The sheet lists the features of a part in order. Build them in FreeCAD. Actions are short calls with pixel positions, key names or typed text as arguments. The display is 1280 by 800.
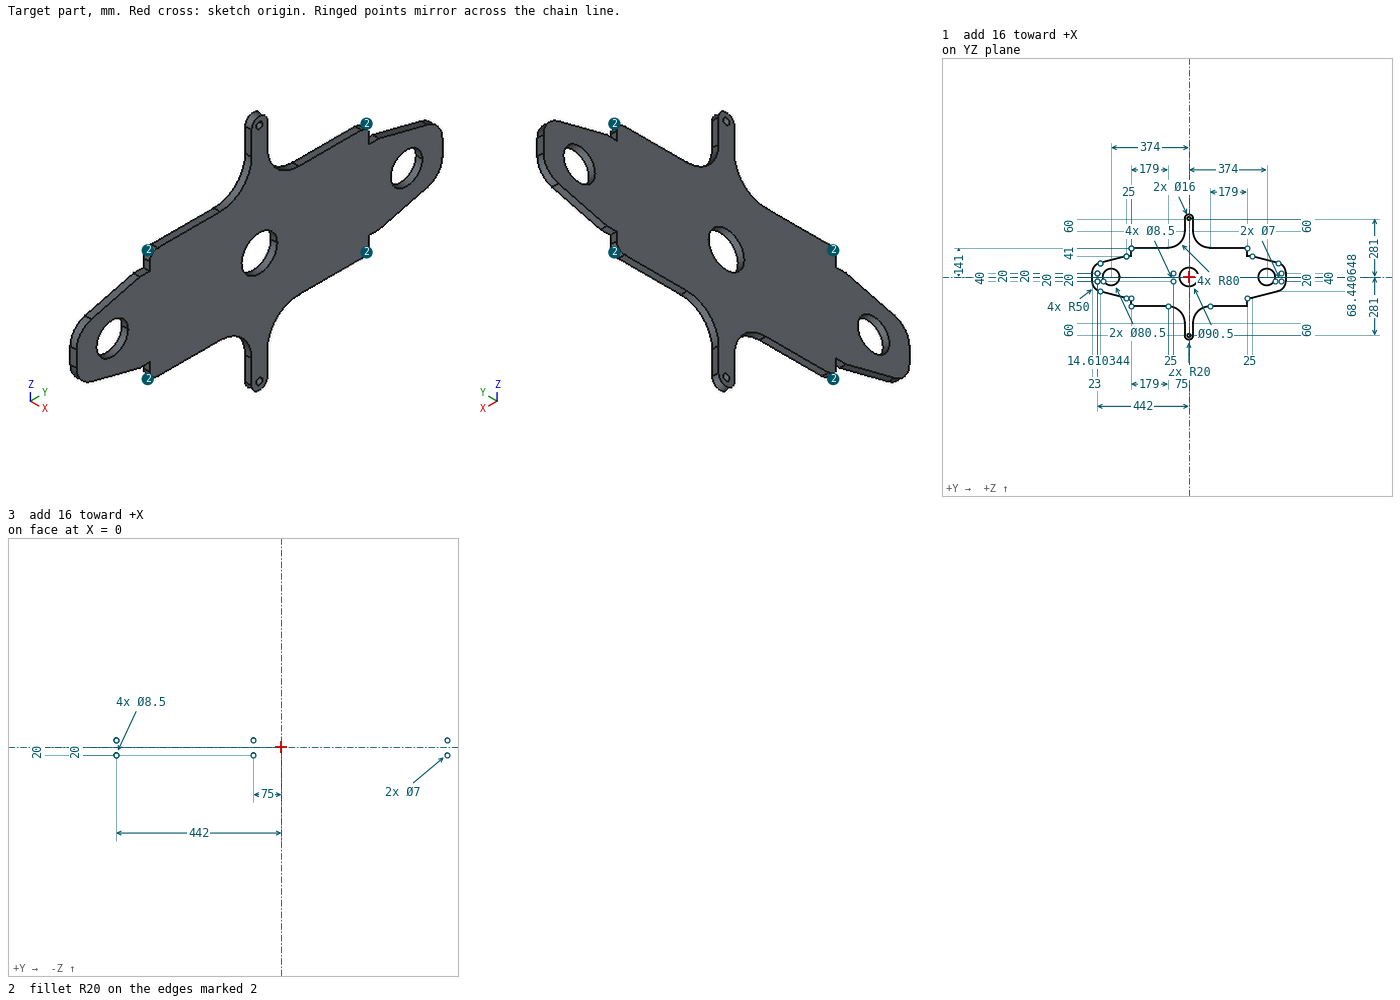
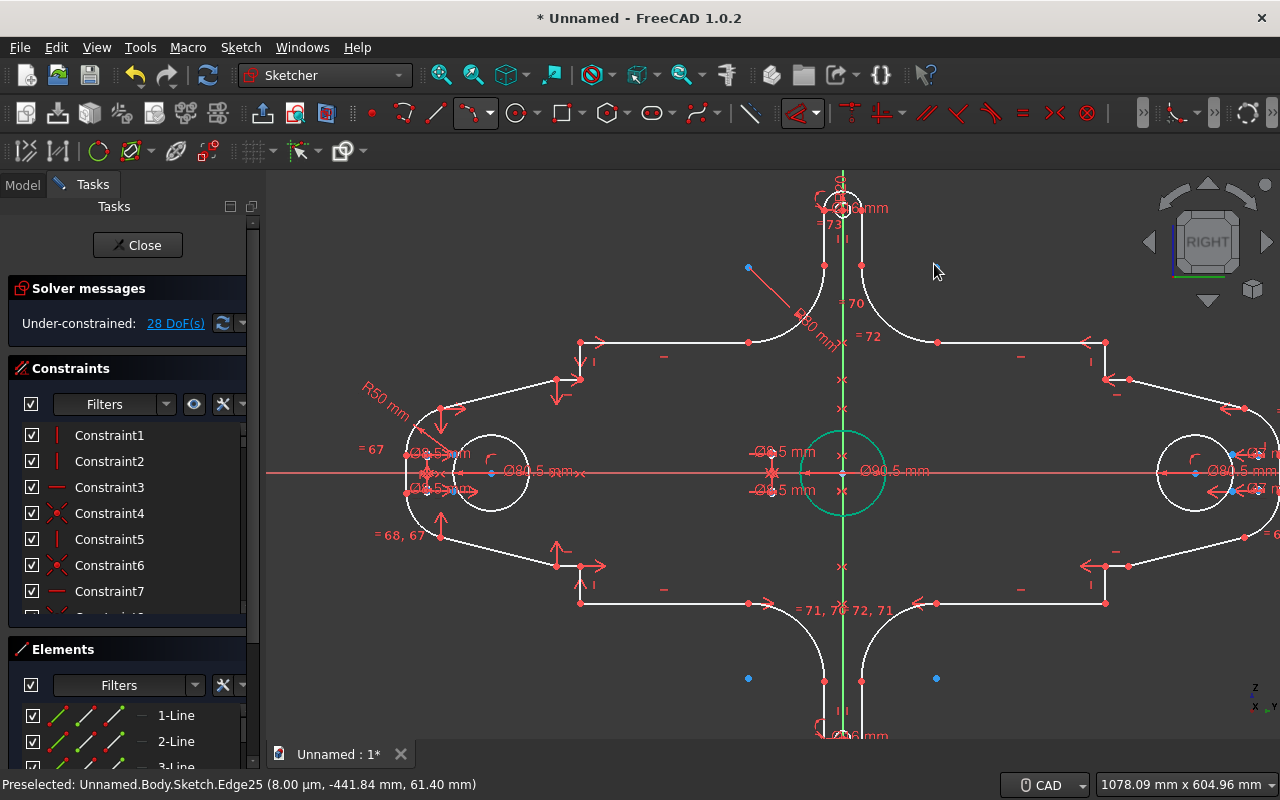
click(862, 249)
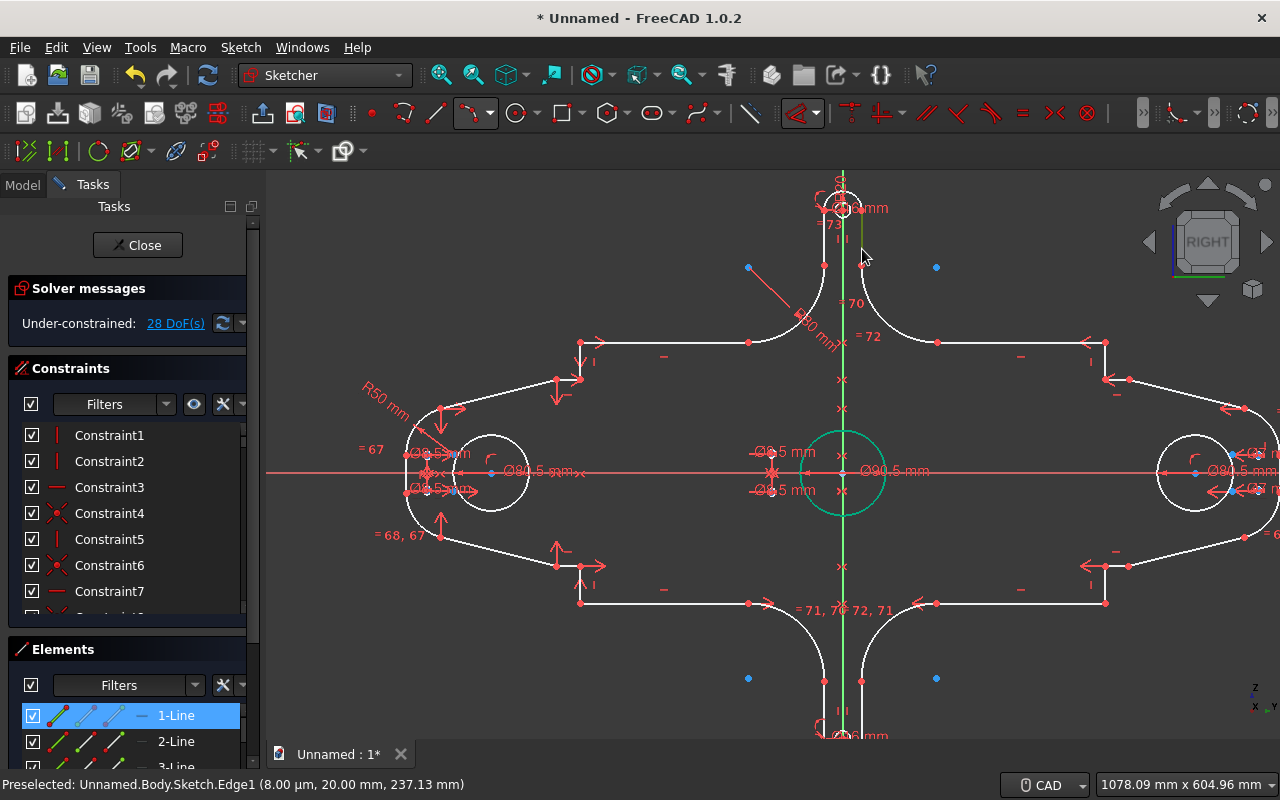
key(i)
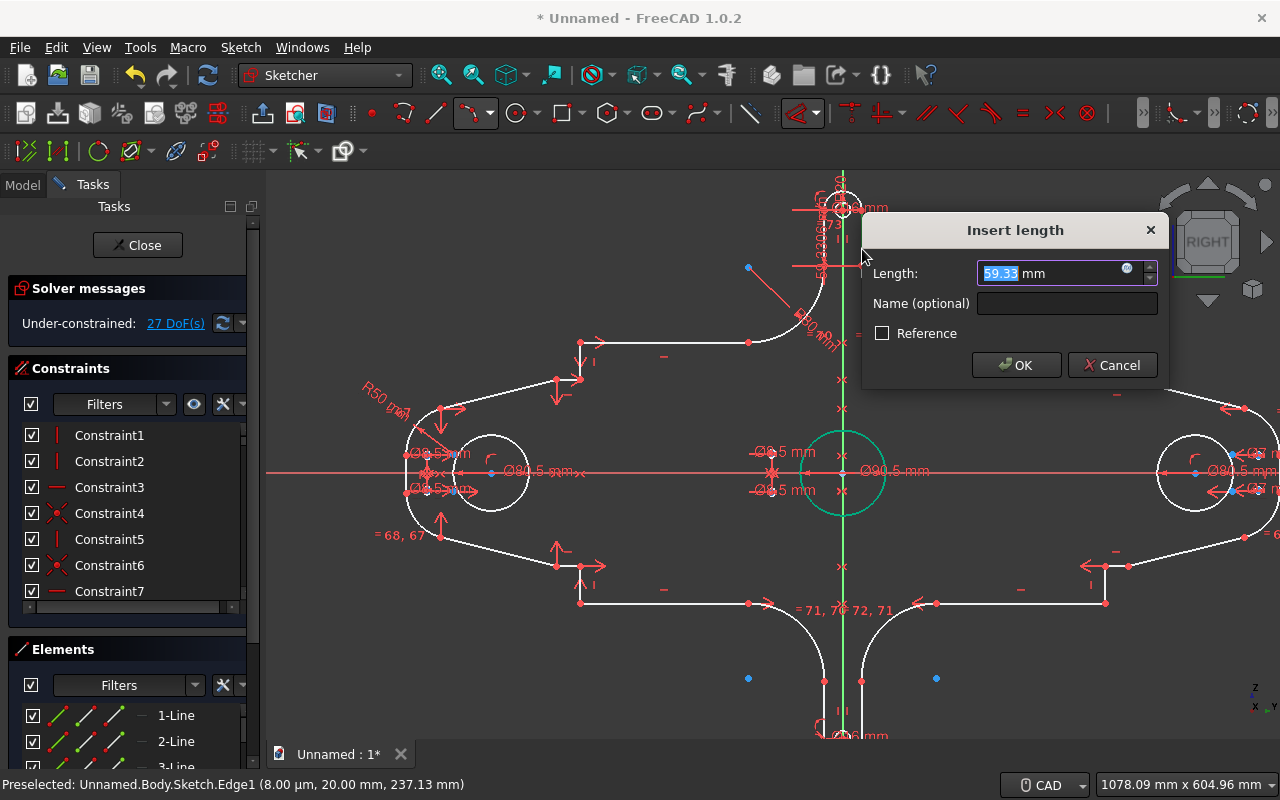
text(60)
key(Return)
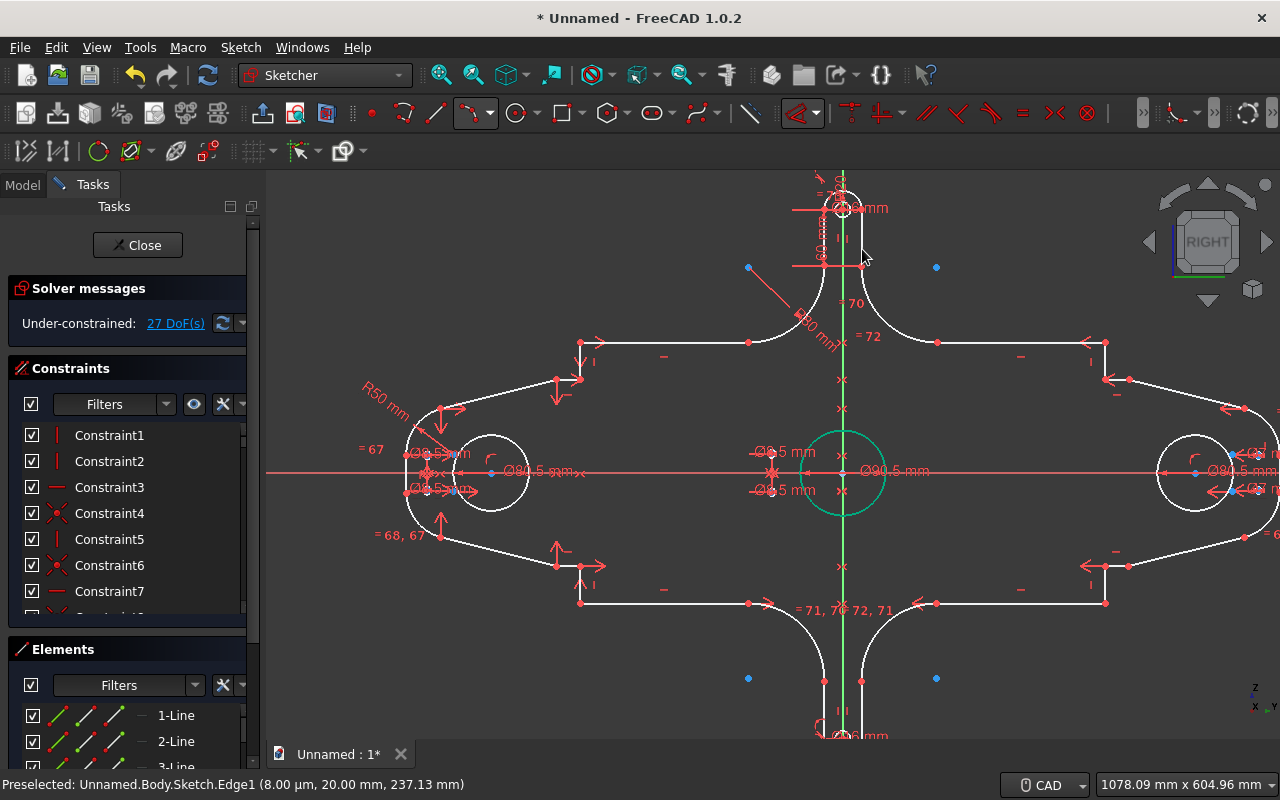
scroll(824, 227, up, 4)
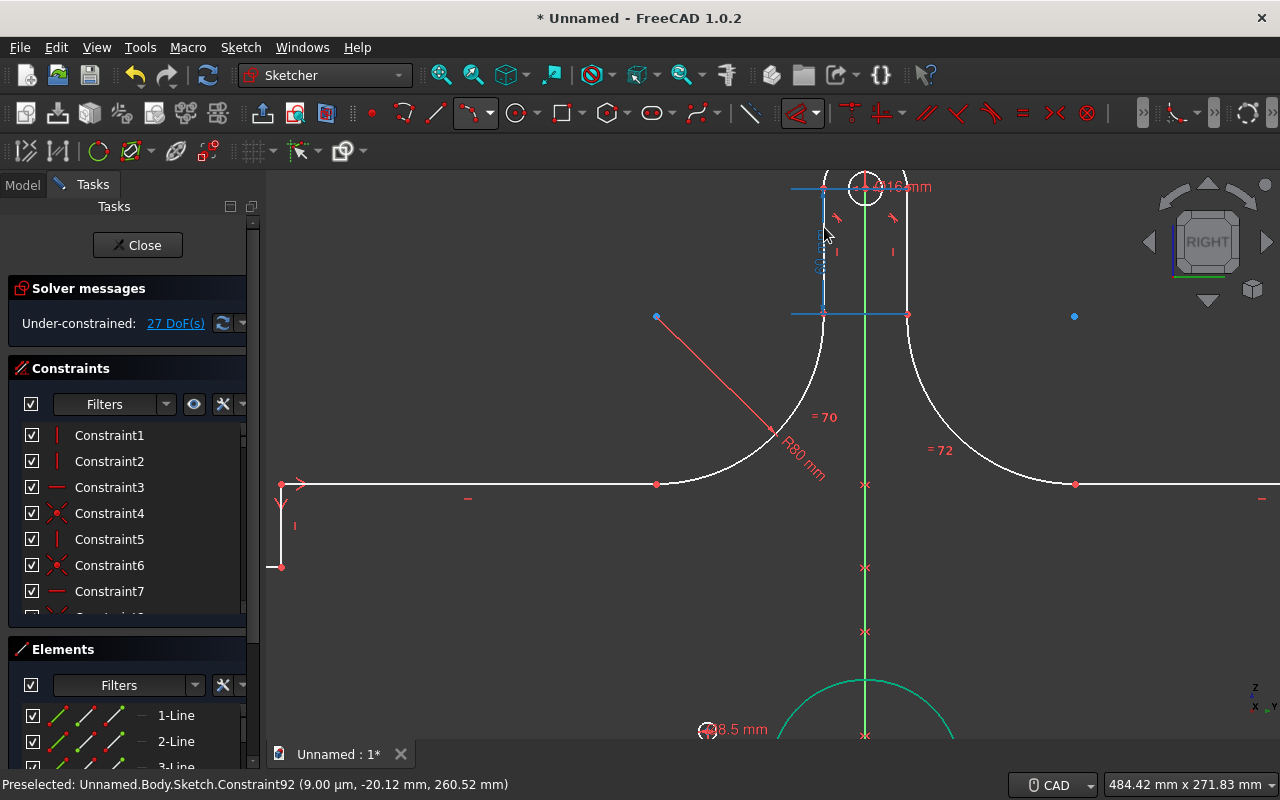
click(824, 226)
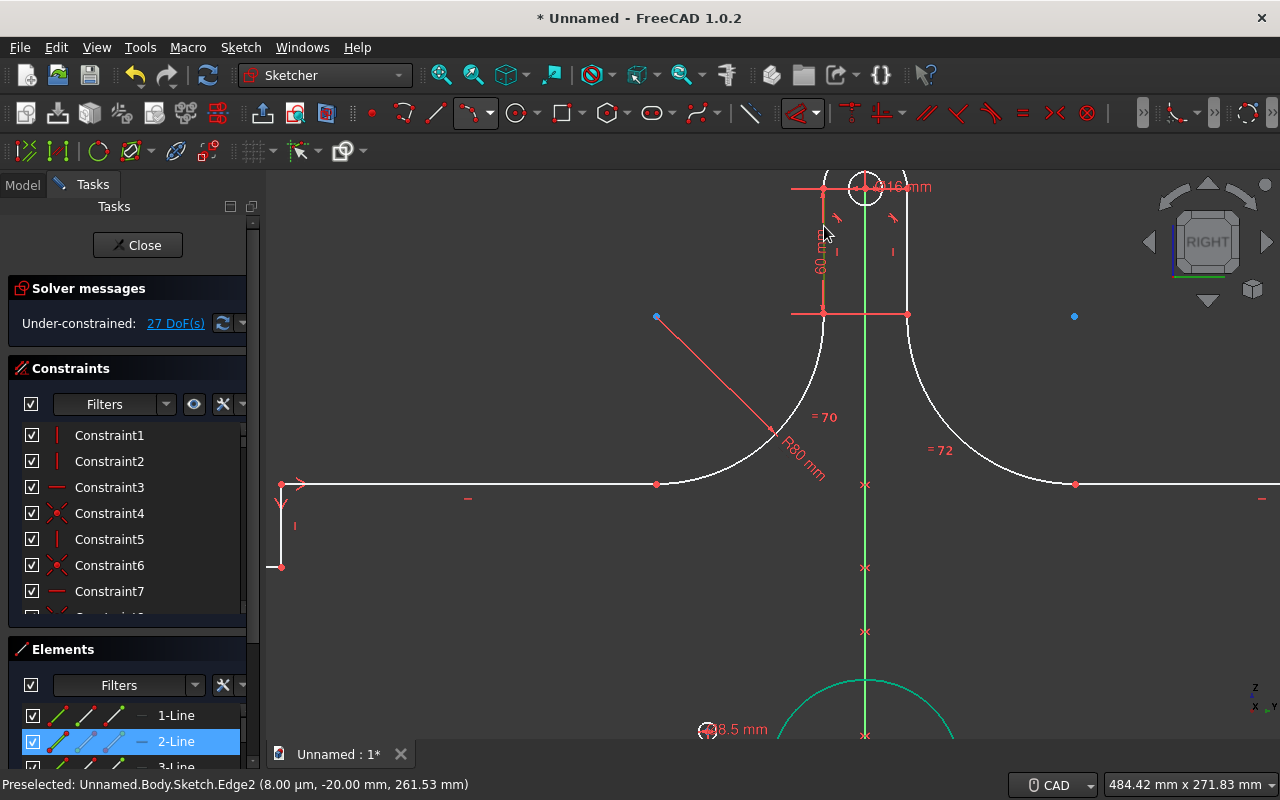
click(818, 114)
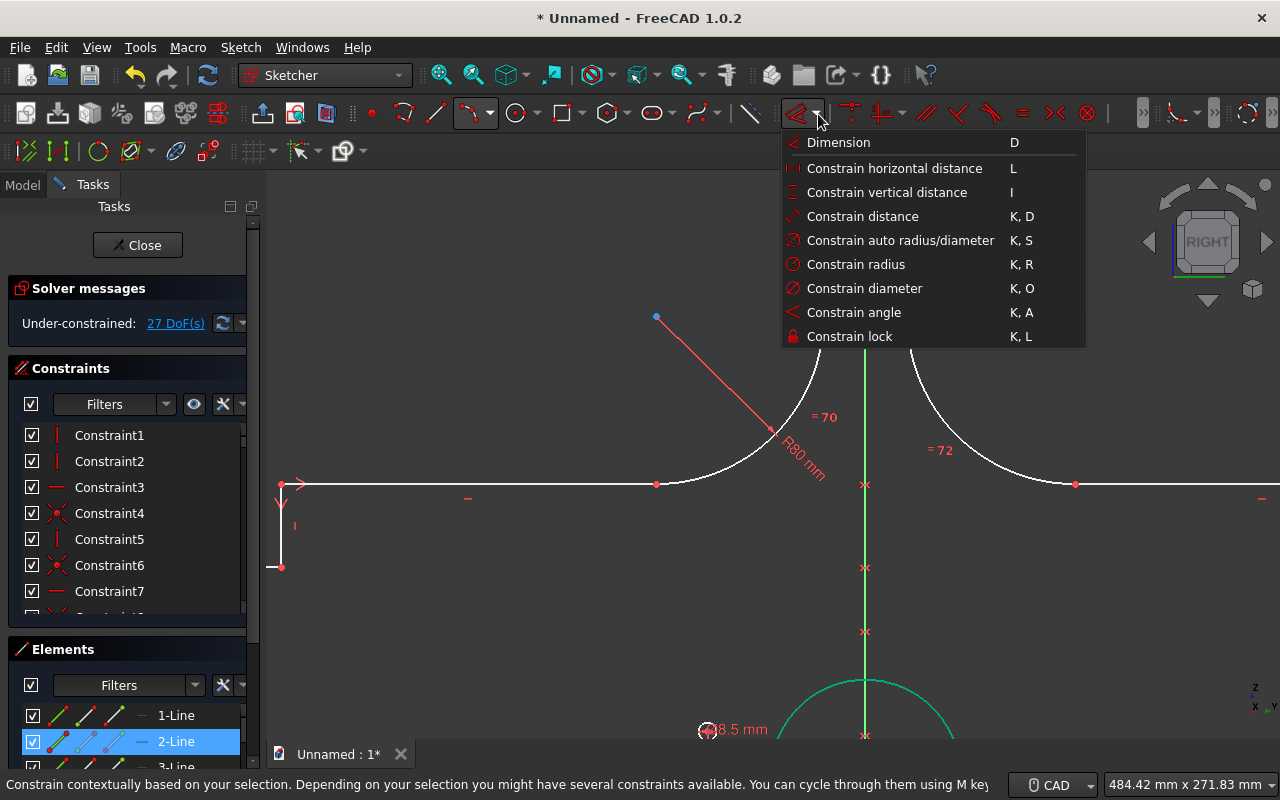
click(934, 192)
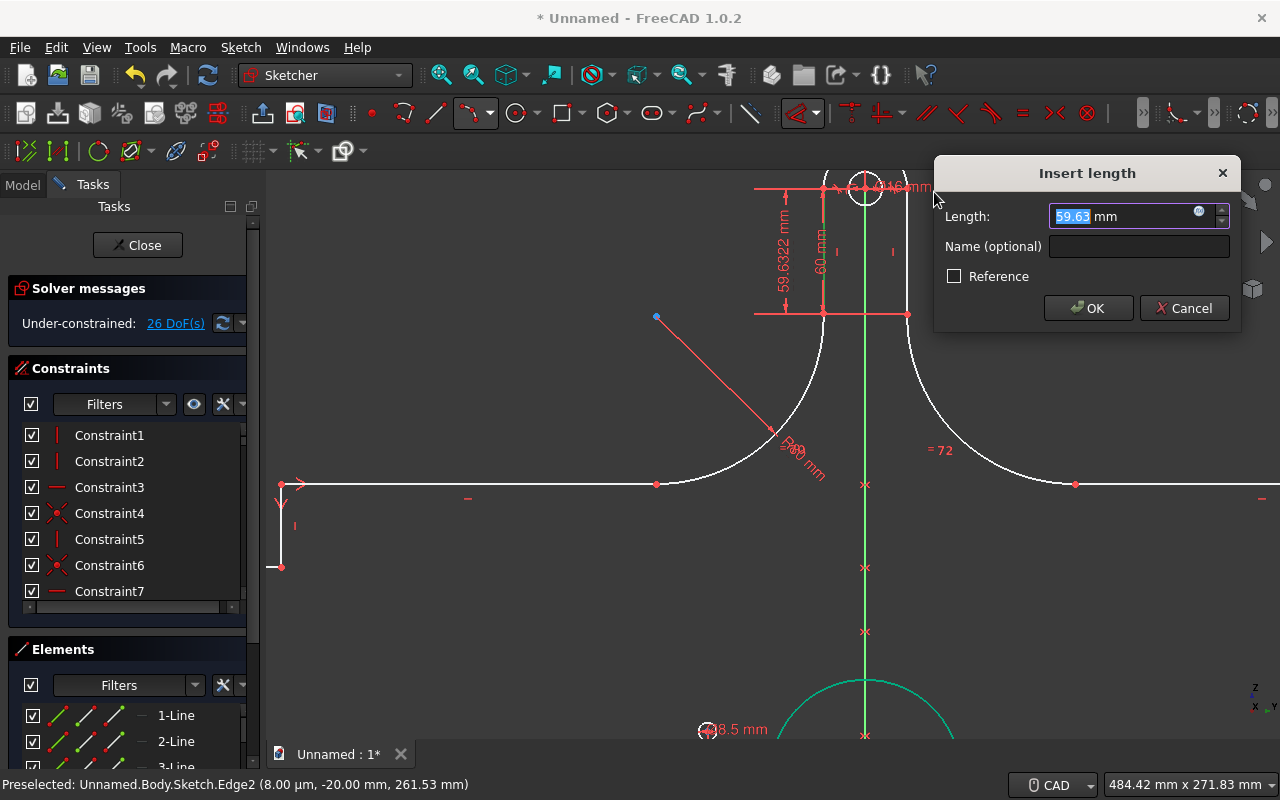
text(60)
key(Return)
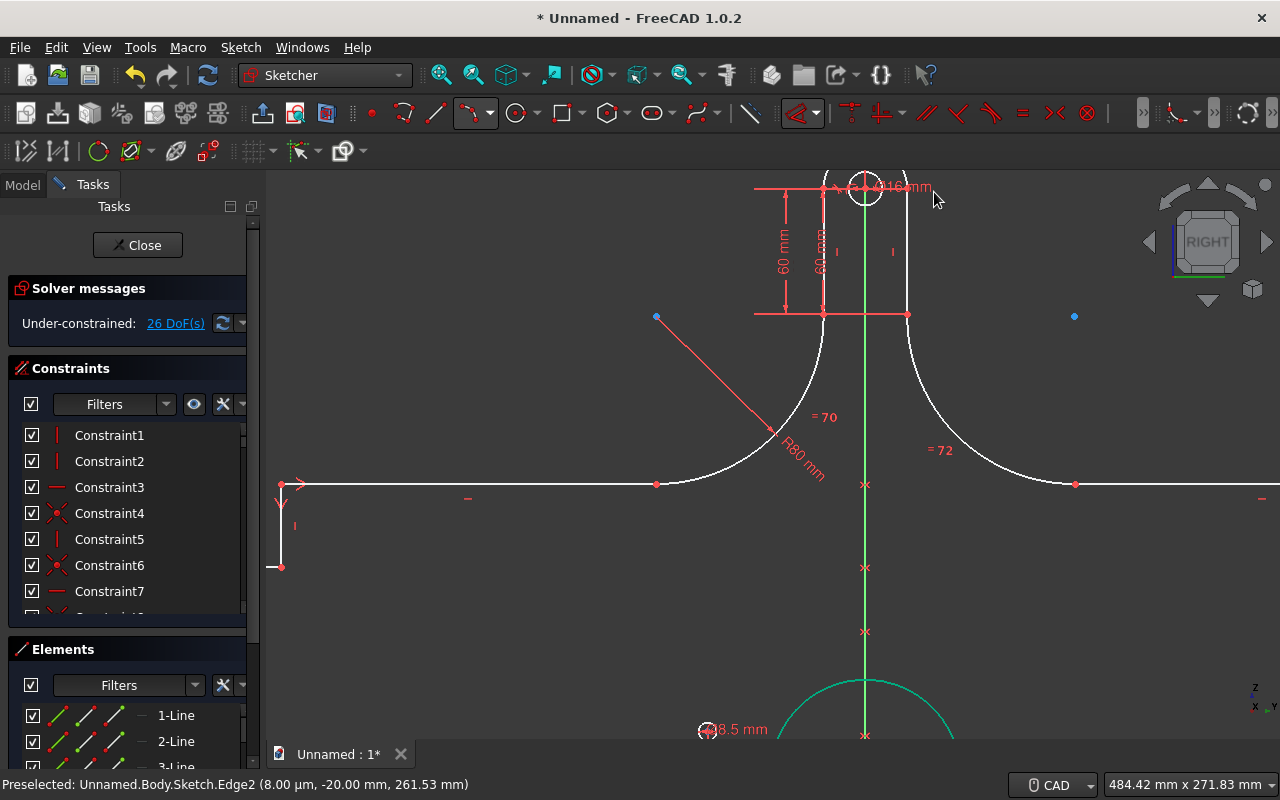
scroll(635, 317, down, 6)